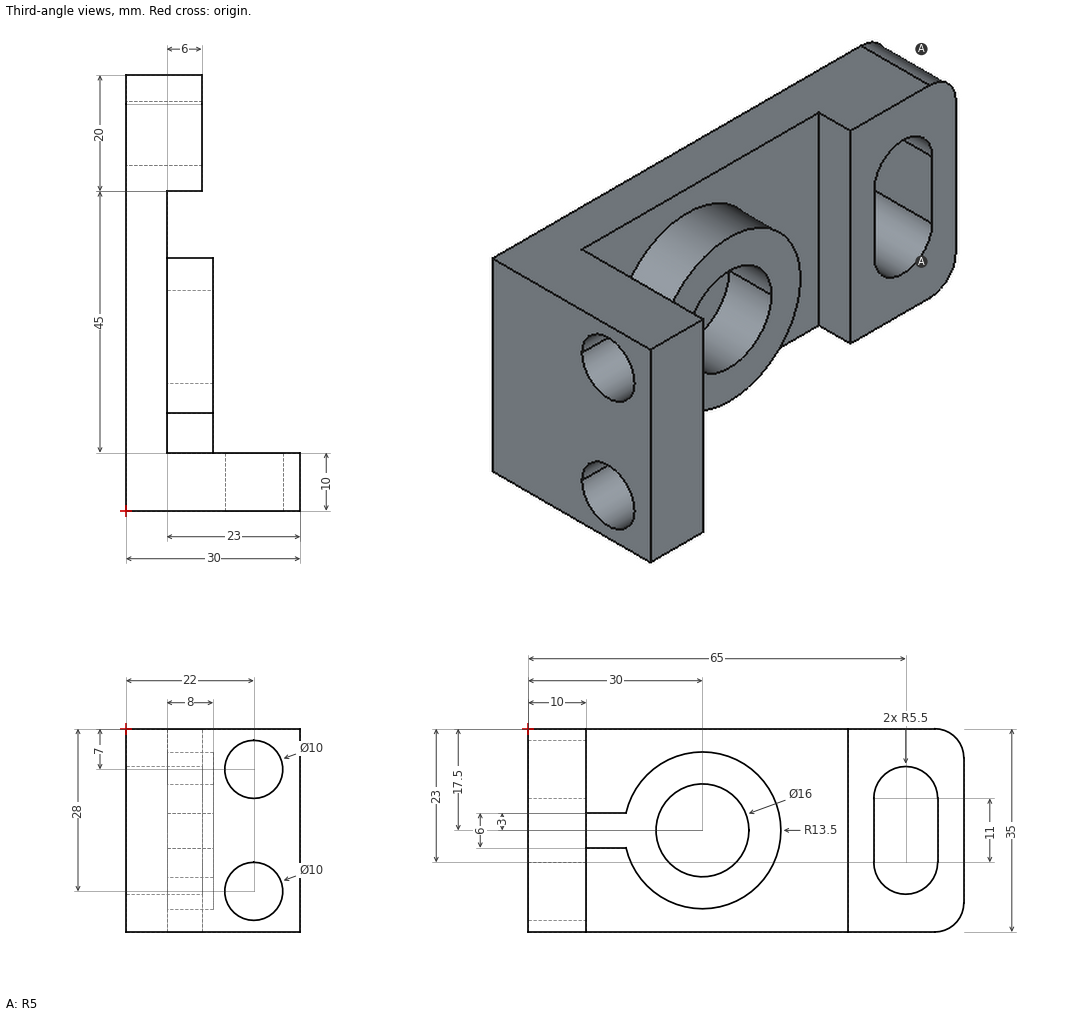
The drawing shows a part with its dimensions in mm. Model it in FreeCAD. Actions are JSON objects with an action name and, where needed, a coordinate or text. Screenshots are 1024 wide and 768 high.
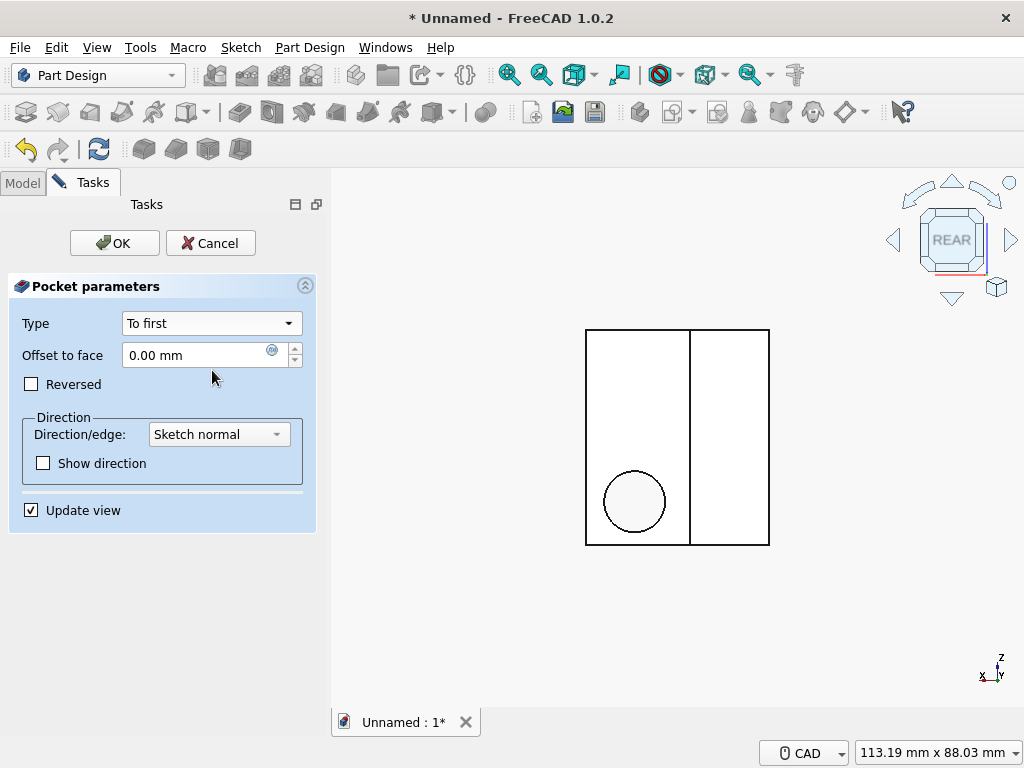
{"action": "left_click", "coordinate": [115, 243]}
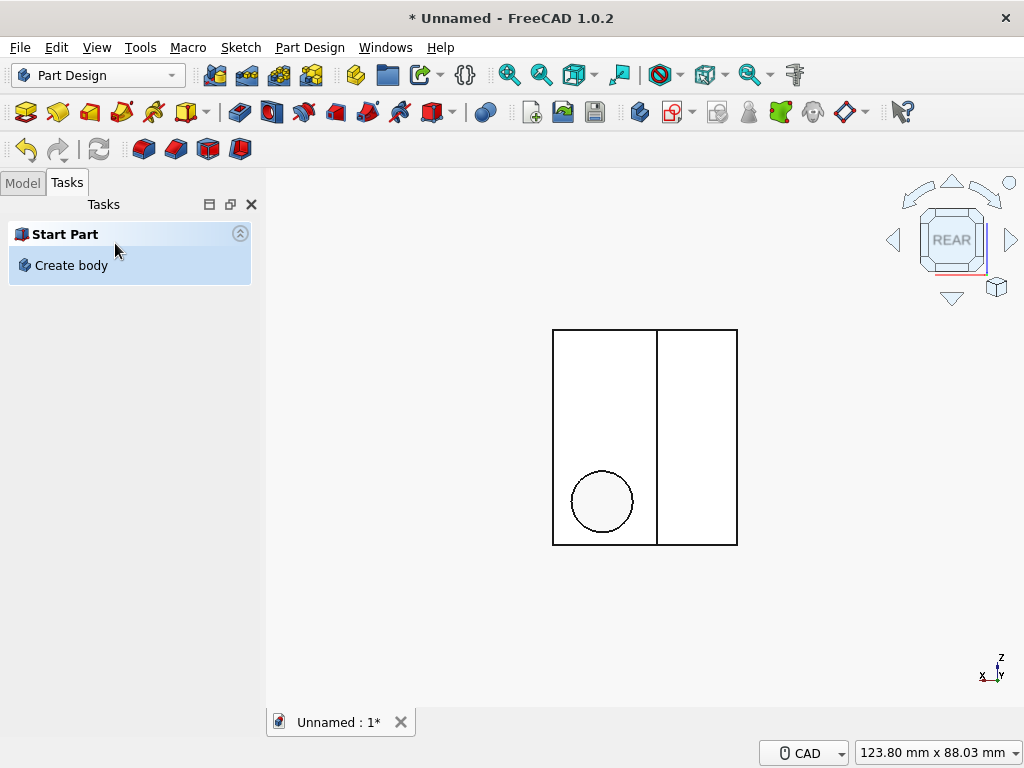
{"action": "left_click", "coordinate": [510, 76]}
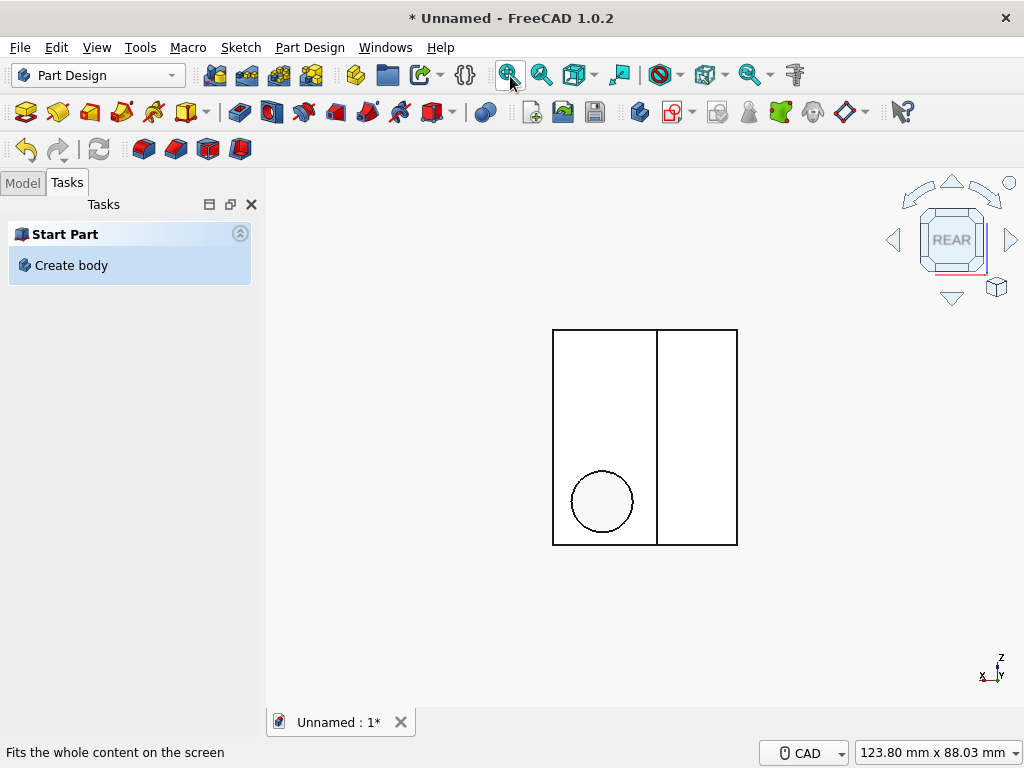
{"action": "left_click", "coordinate": [624, 406]}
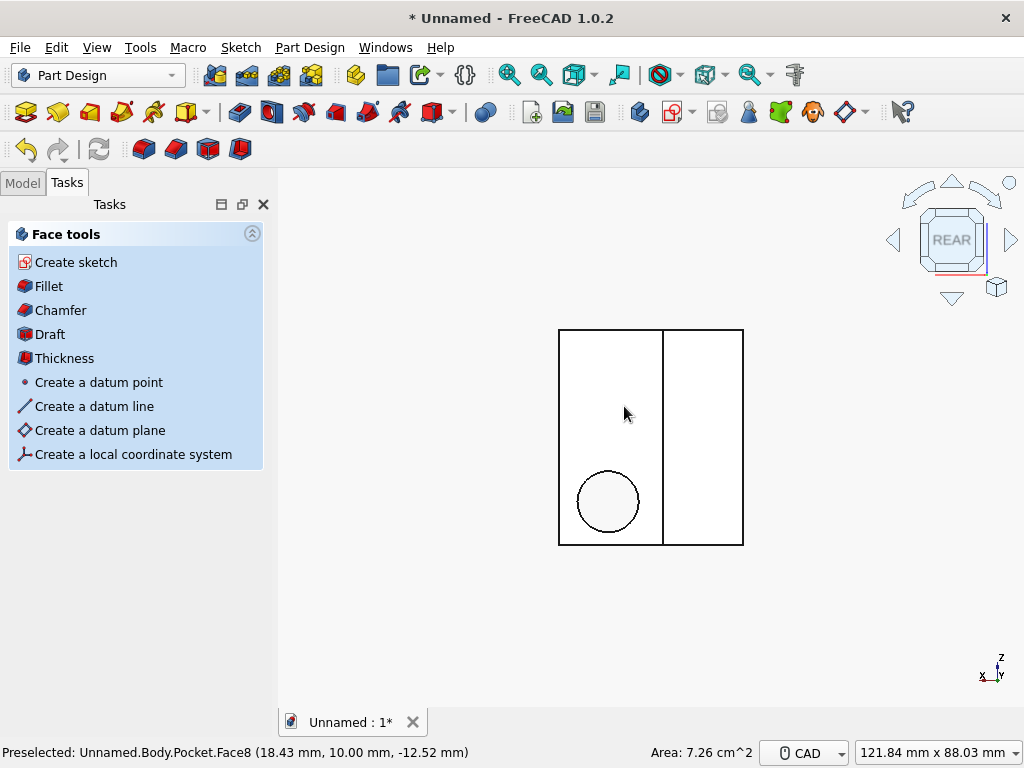
{"action": "left_click", "coordinate": [672, 112]}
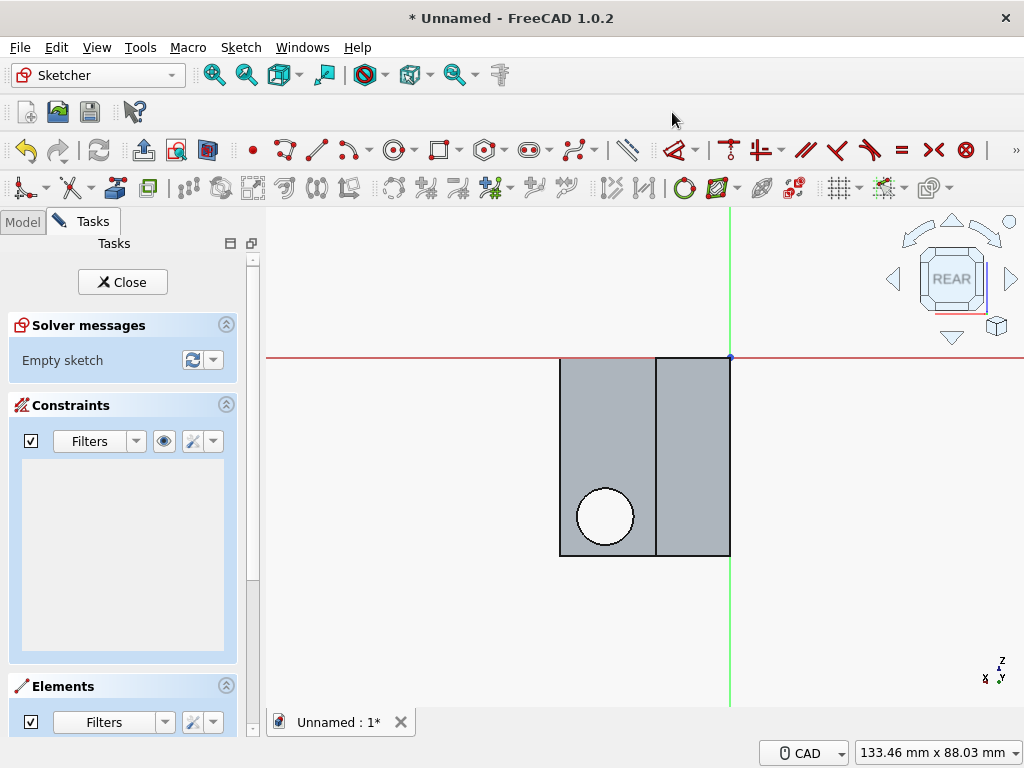
{"action": "key", "text": "q s"}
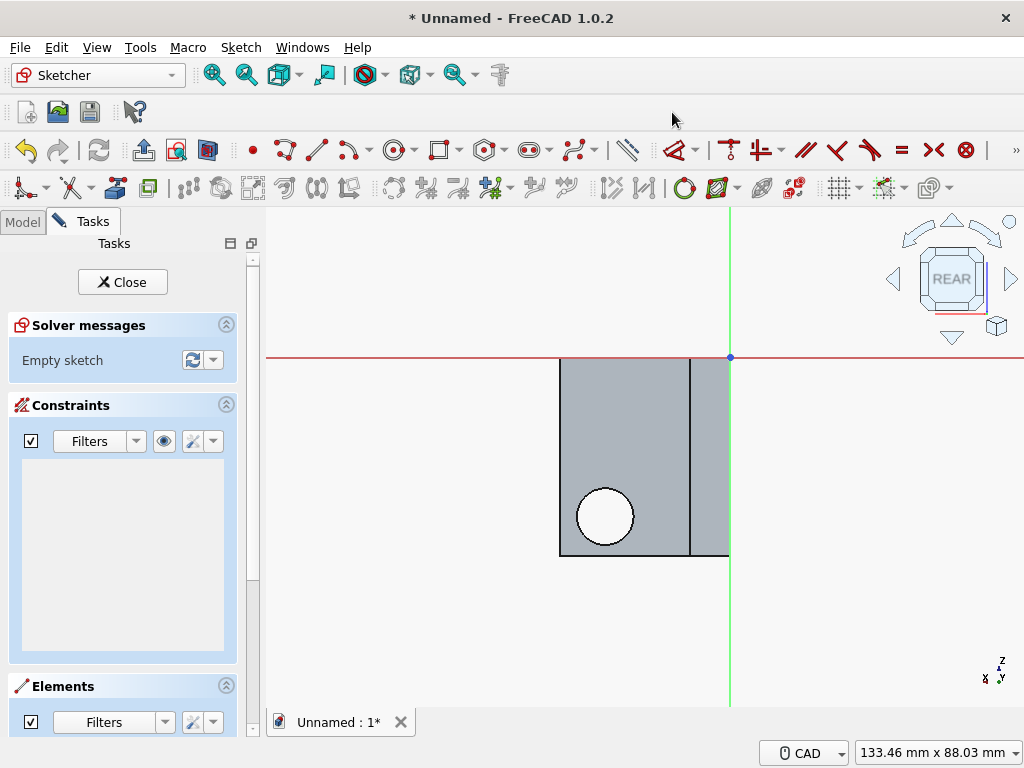
{"action": "scroll", "coordinate": [611, 386], "scroll_direction": "up", "scroll_amount": 9}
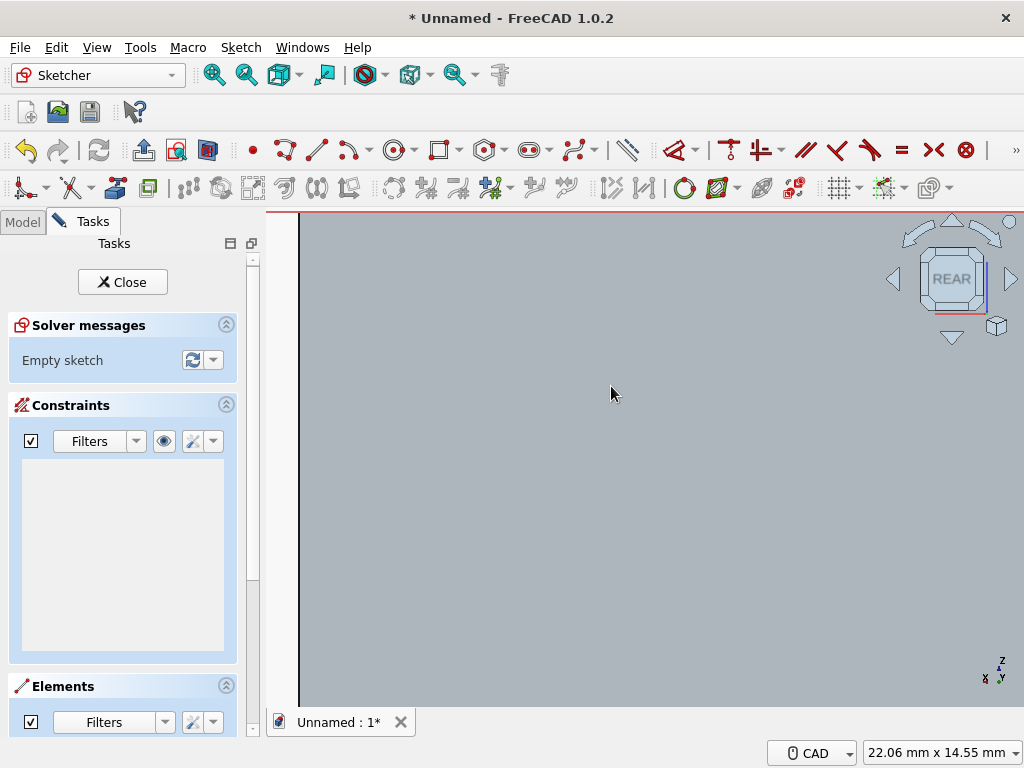
{"action": "left_click", "coordinate": [394, 150]}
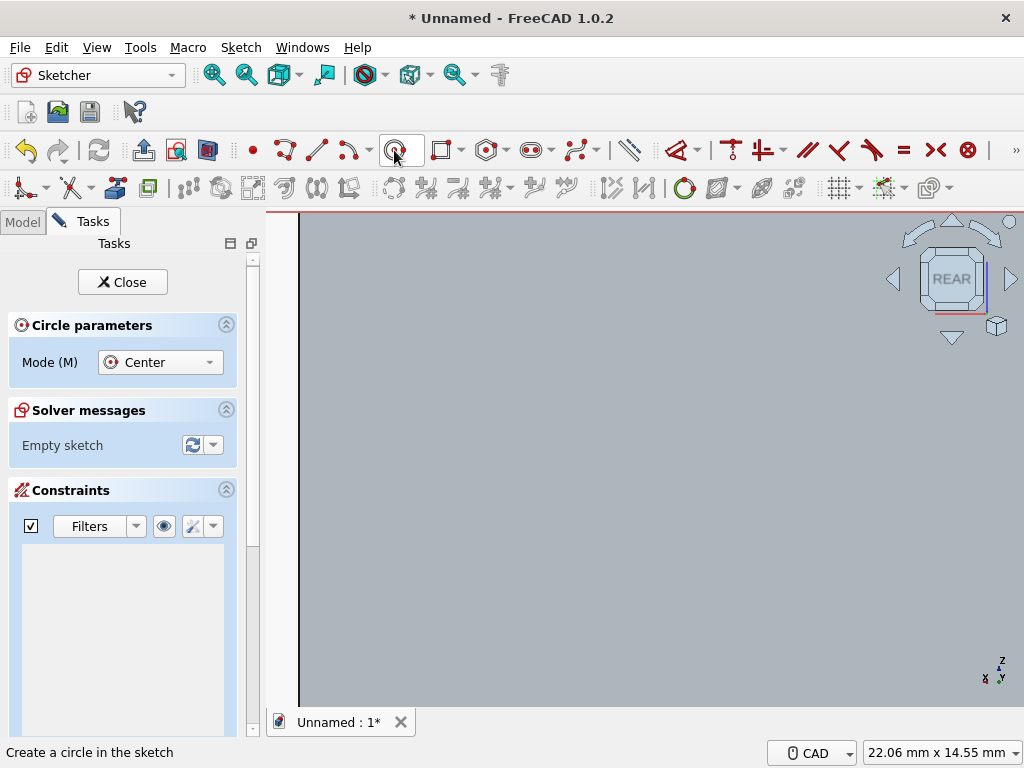
{"action": "left_click", "coordinate": [574, 453]}
{"action": "left_click", "coordinate": [695, 331]}
{"action": "key", "text": "Escape"}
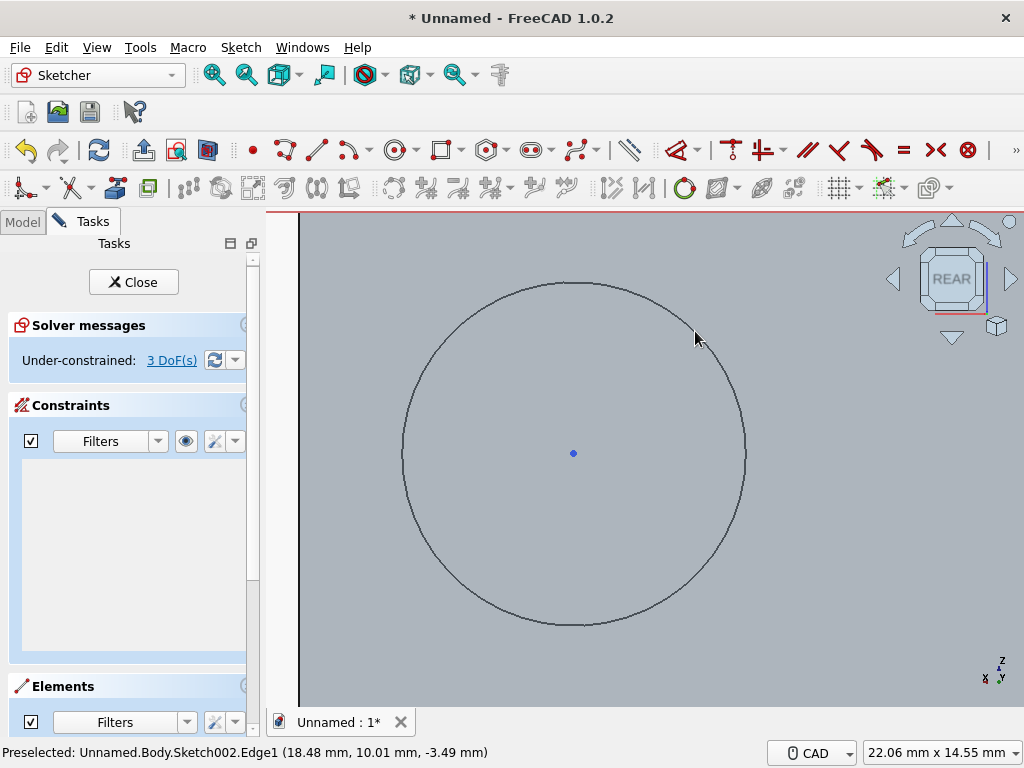
{"action": "left_click", "coordinate": [676, 150]}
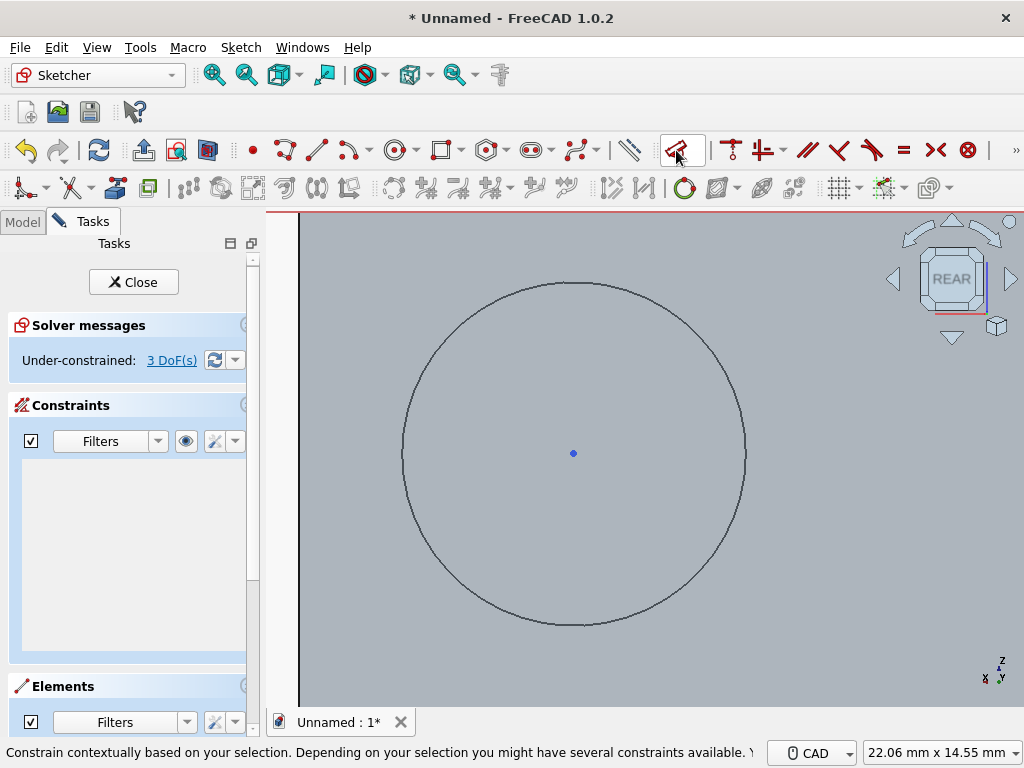
{"action": "left_click", "coordinate": [695, 332]}
{"action": "left_click", "coordinate": [718, 309]}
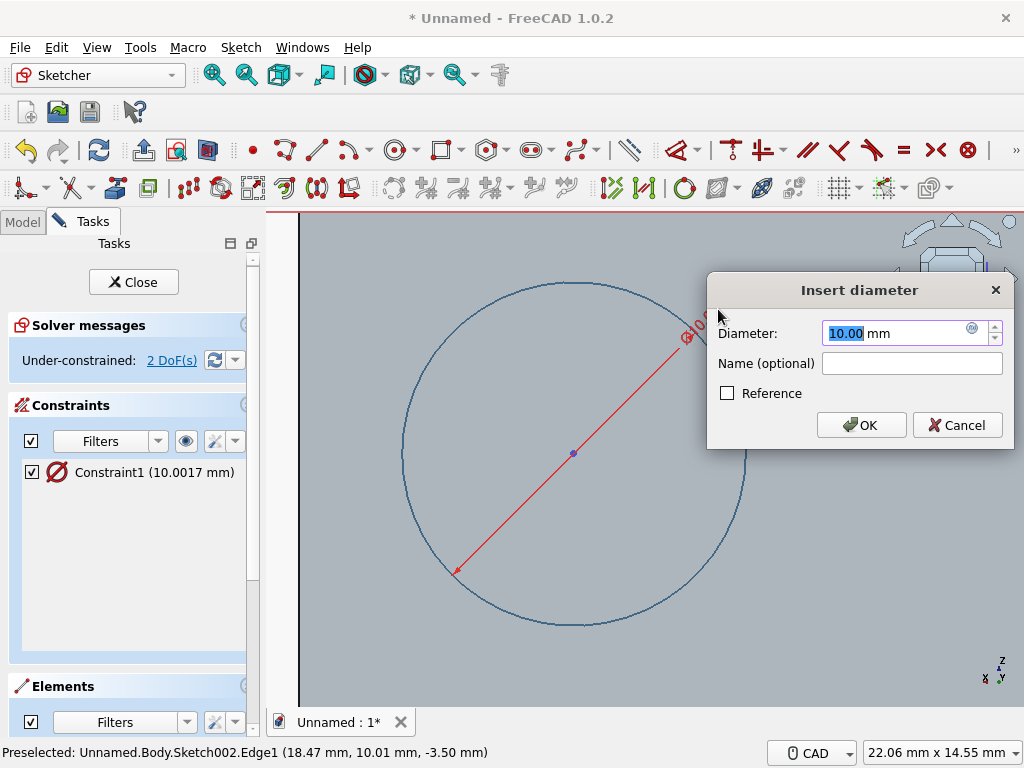
{"action": "type", "text": "10"}
{"action": "key", "text": "Return"}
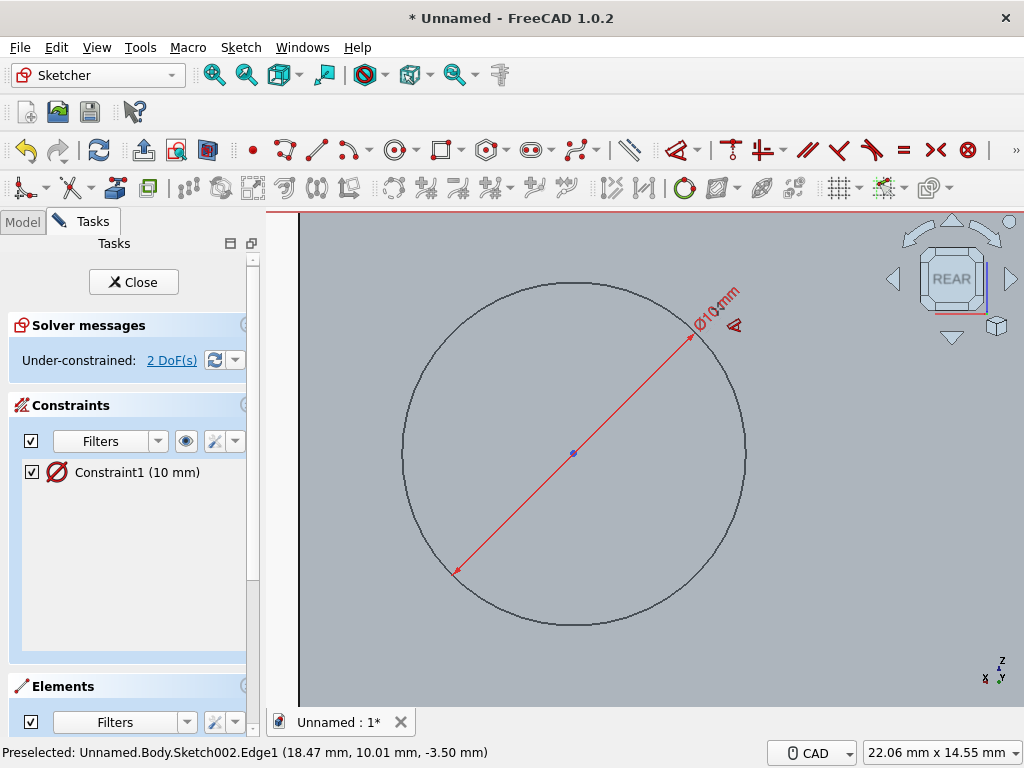
{"action": "left_click", "coordinate": [574, 454]}
{"action": "left_click", "coordinate": [540, 345]}